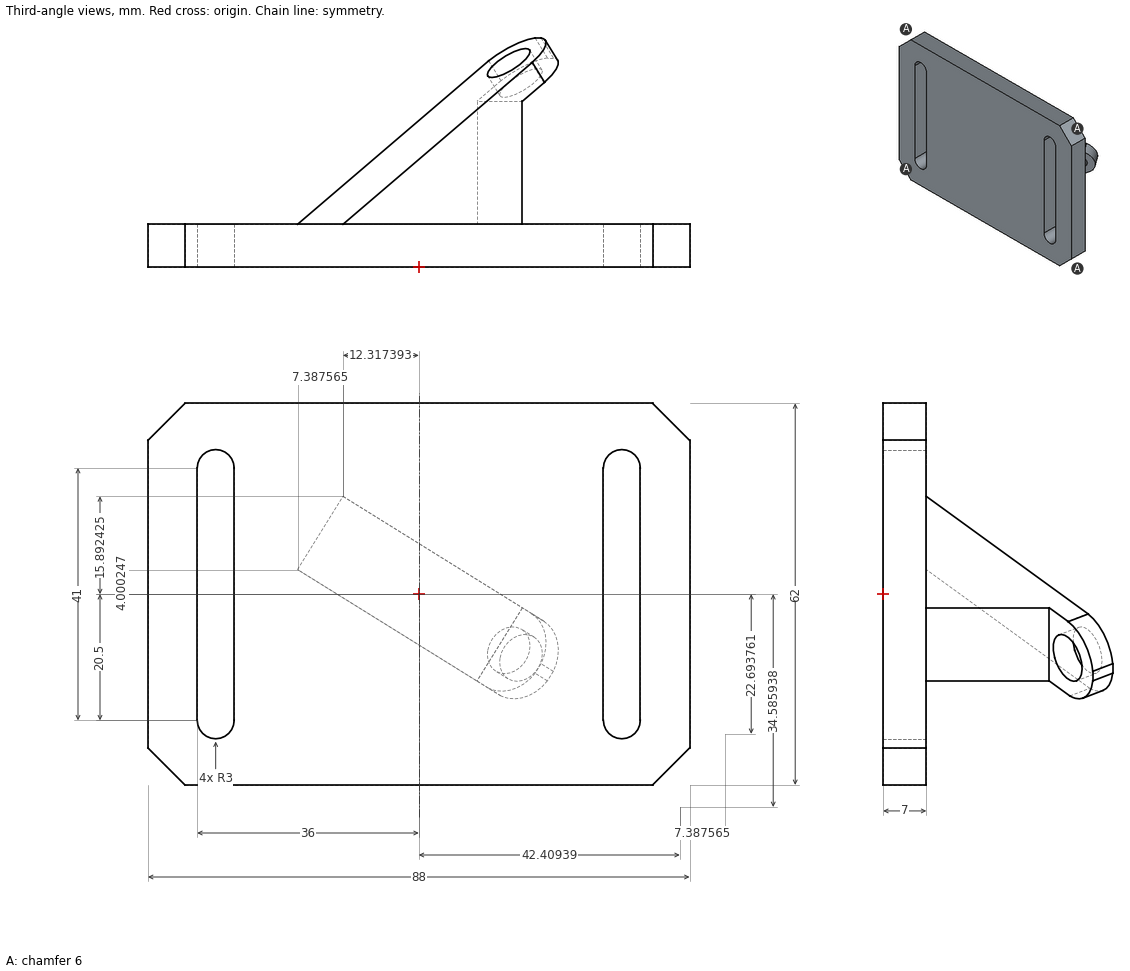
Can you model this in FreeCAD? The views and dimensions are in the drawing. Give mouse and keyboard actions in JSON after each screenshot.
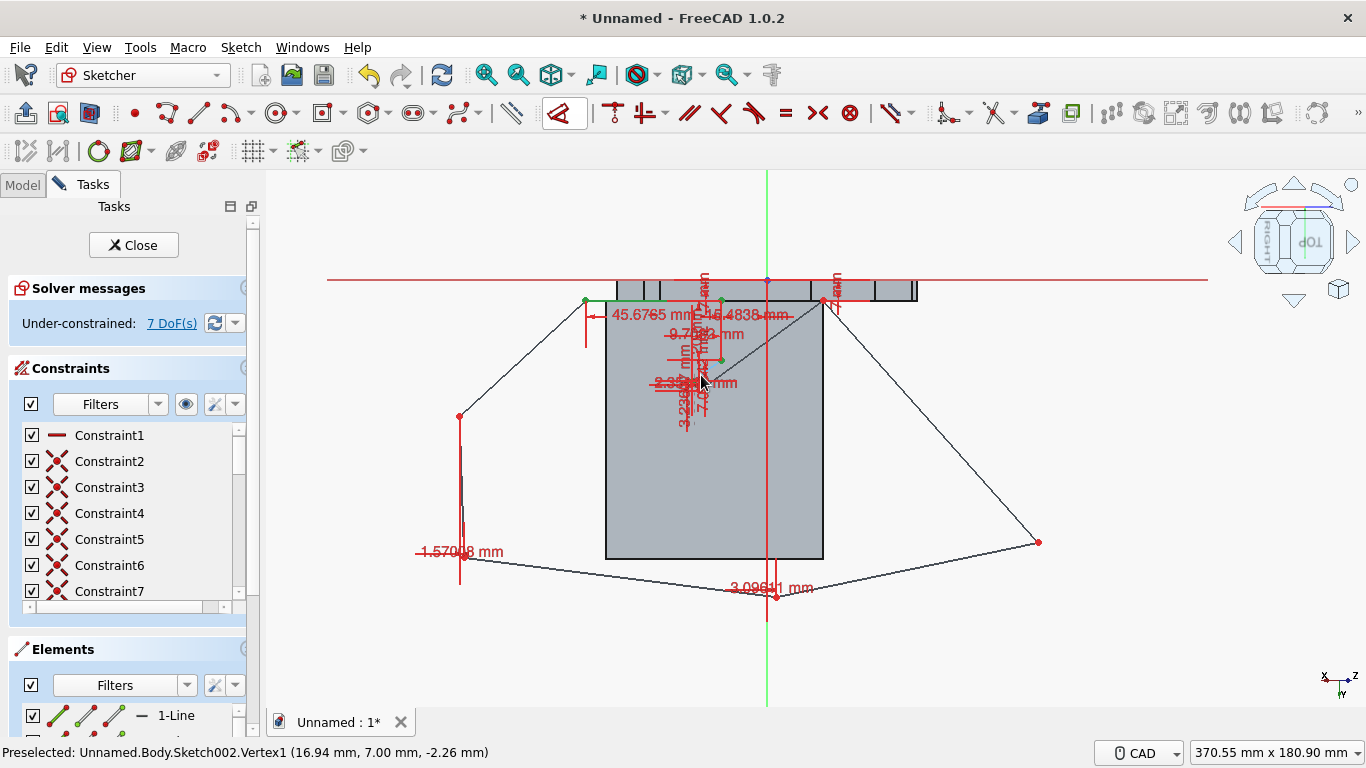
{"action": "left_click", "coordinate": [460, 417]}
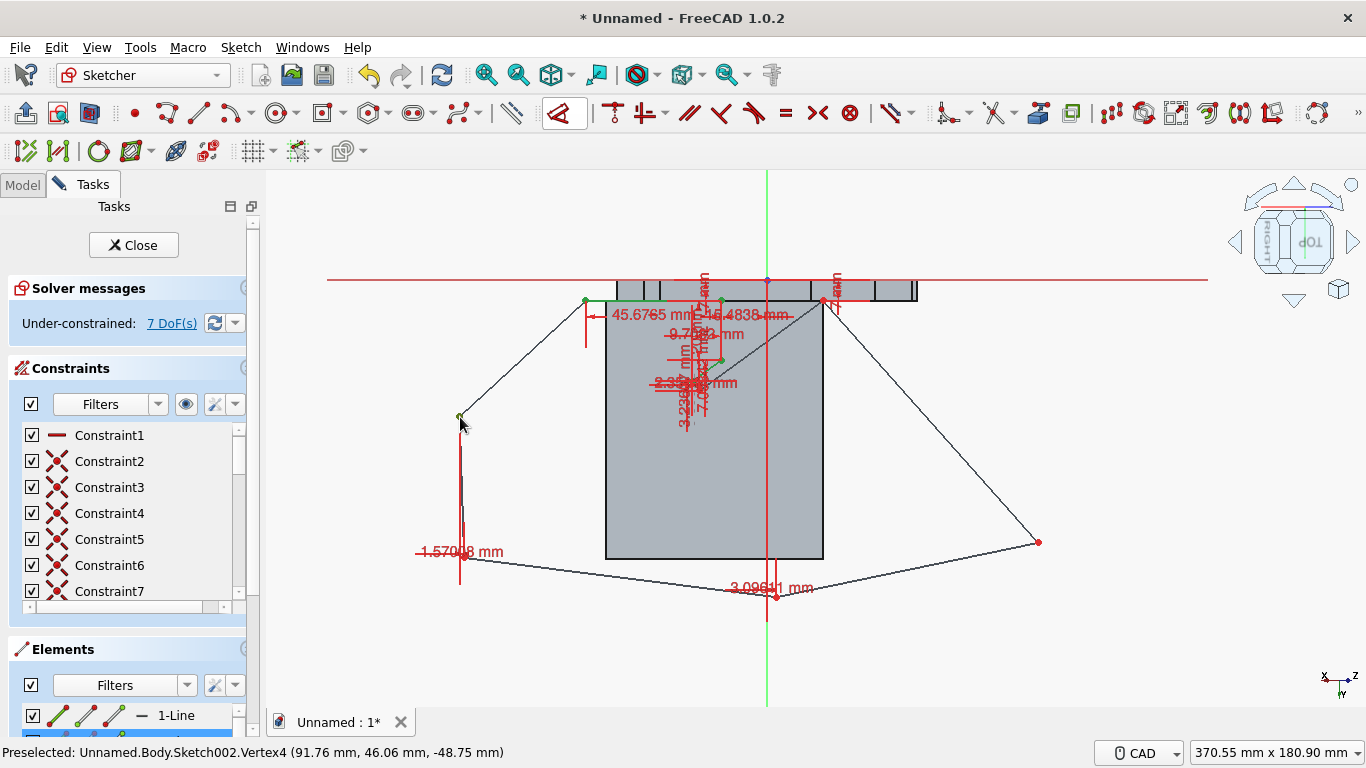
{"action": "left_click", "coordinate": [582, 114]}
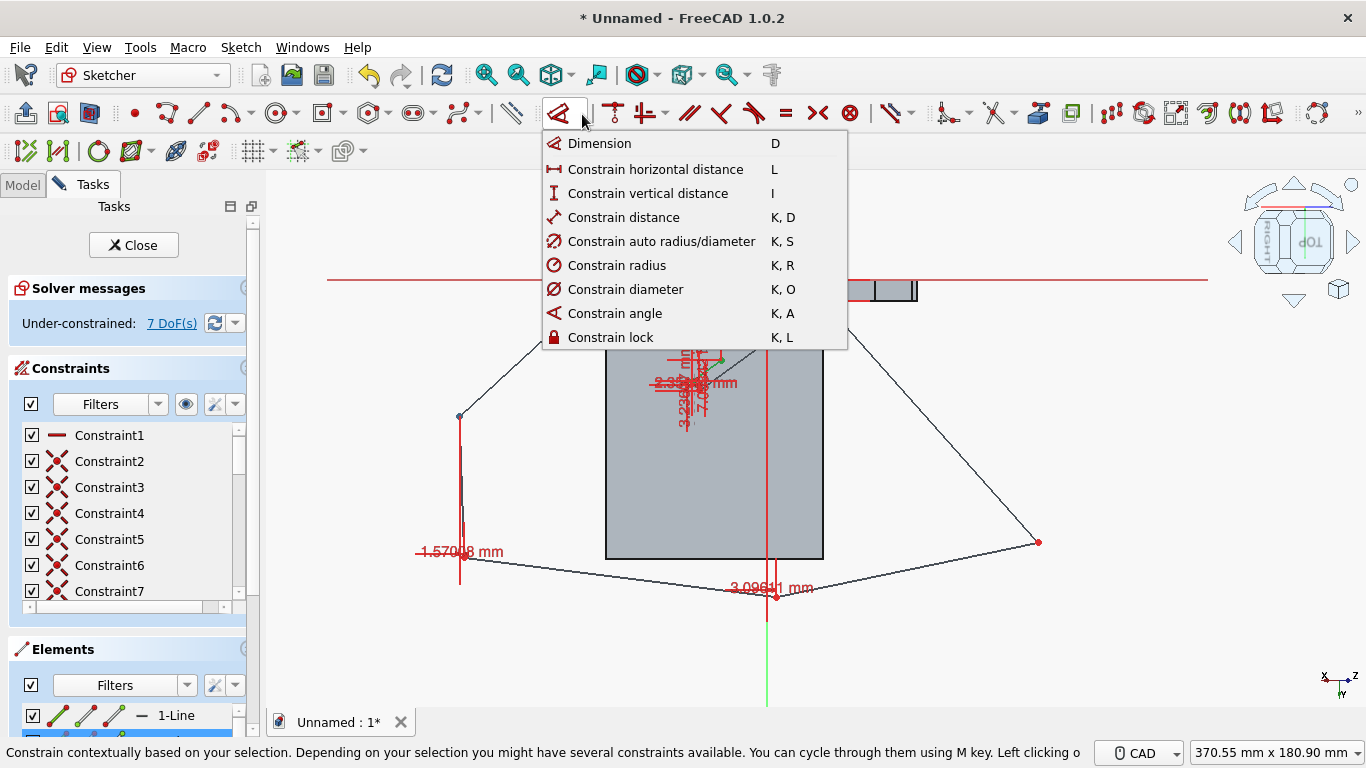
{"action": "left_click", "coordinate": [695, 193]}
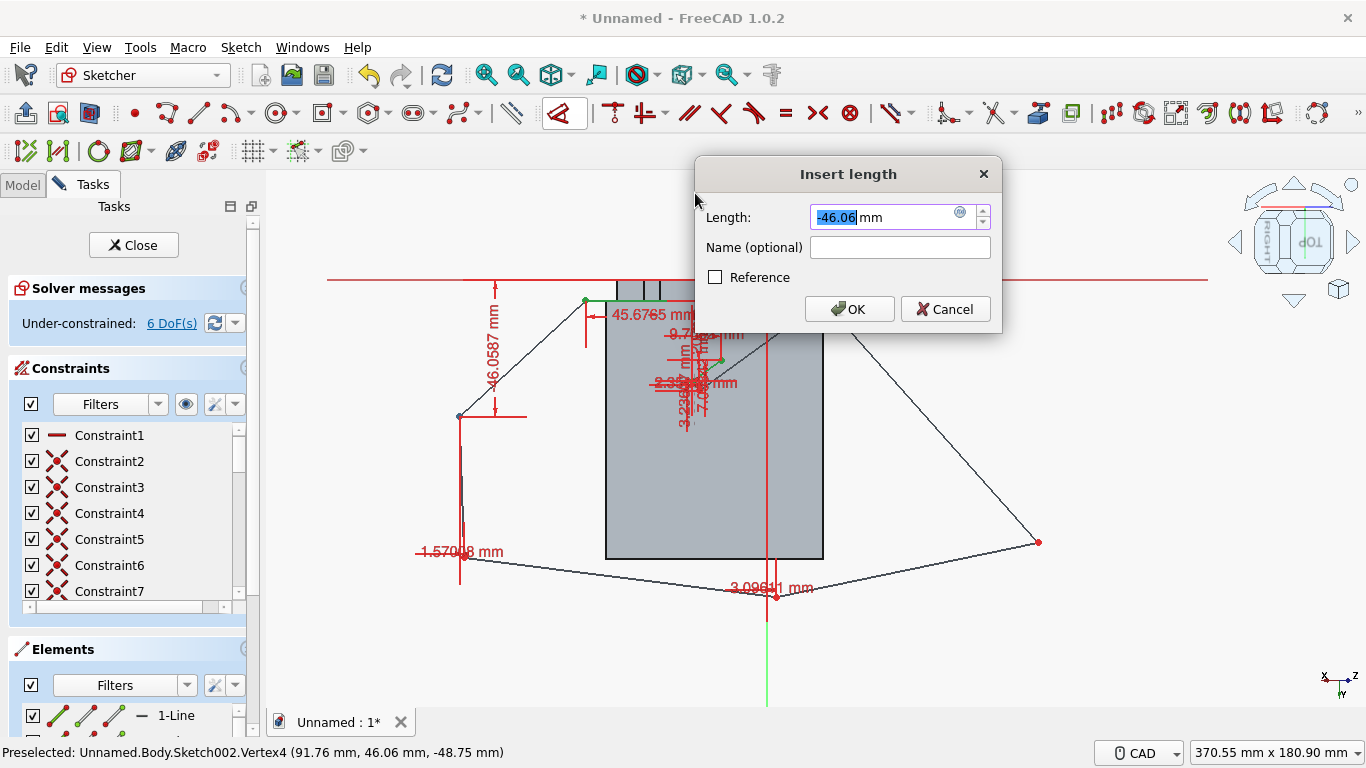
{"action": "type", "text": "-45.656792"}
{"action": "key", "text": "Return"}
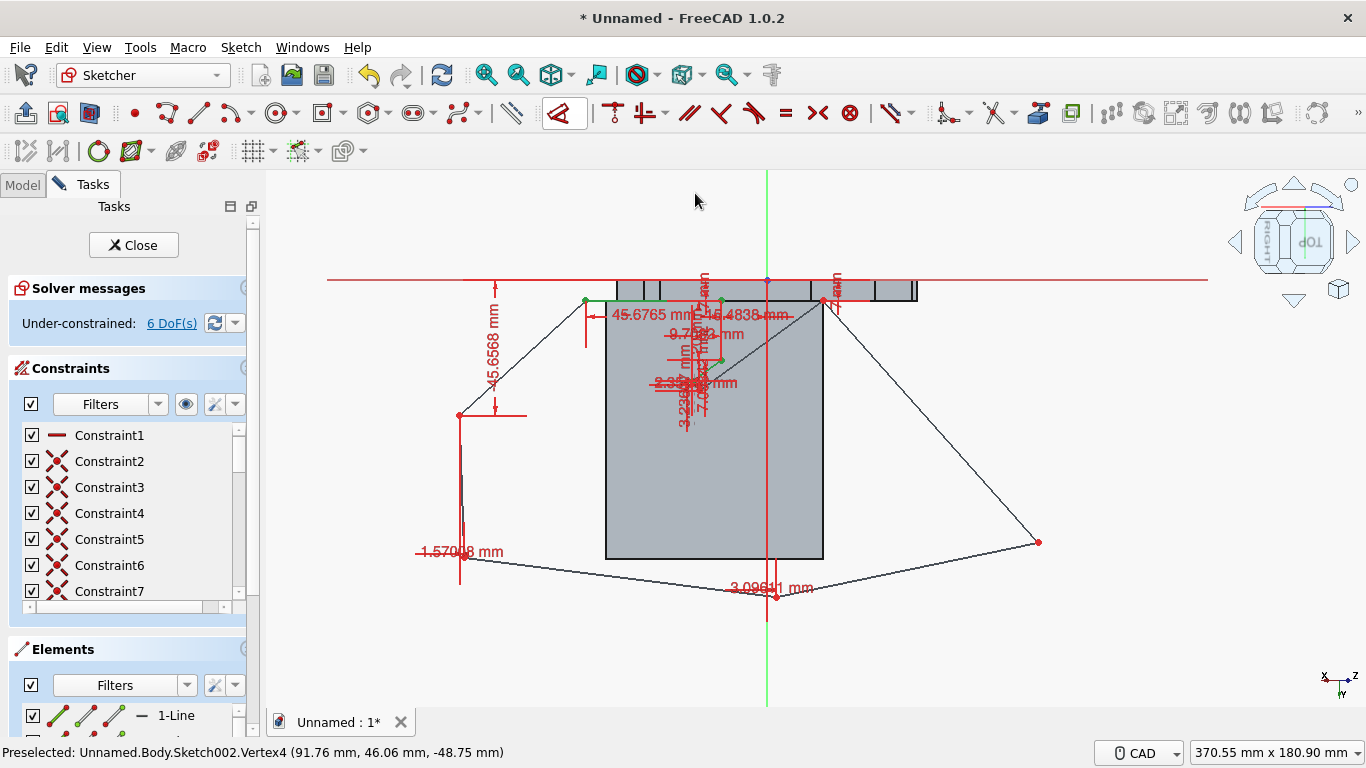
{"action": "left_click", "coordinate": [464, 558]}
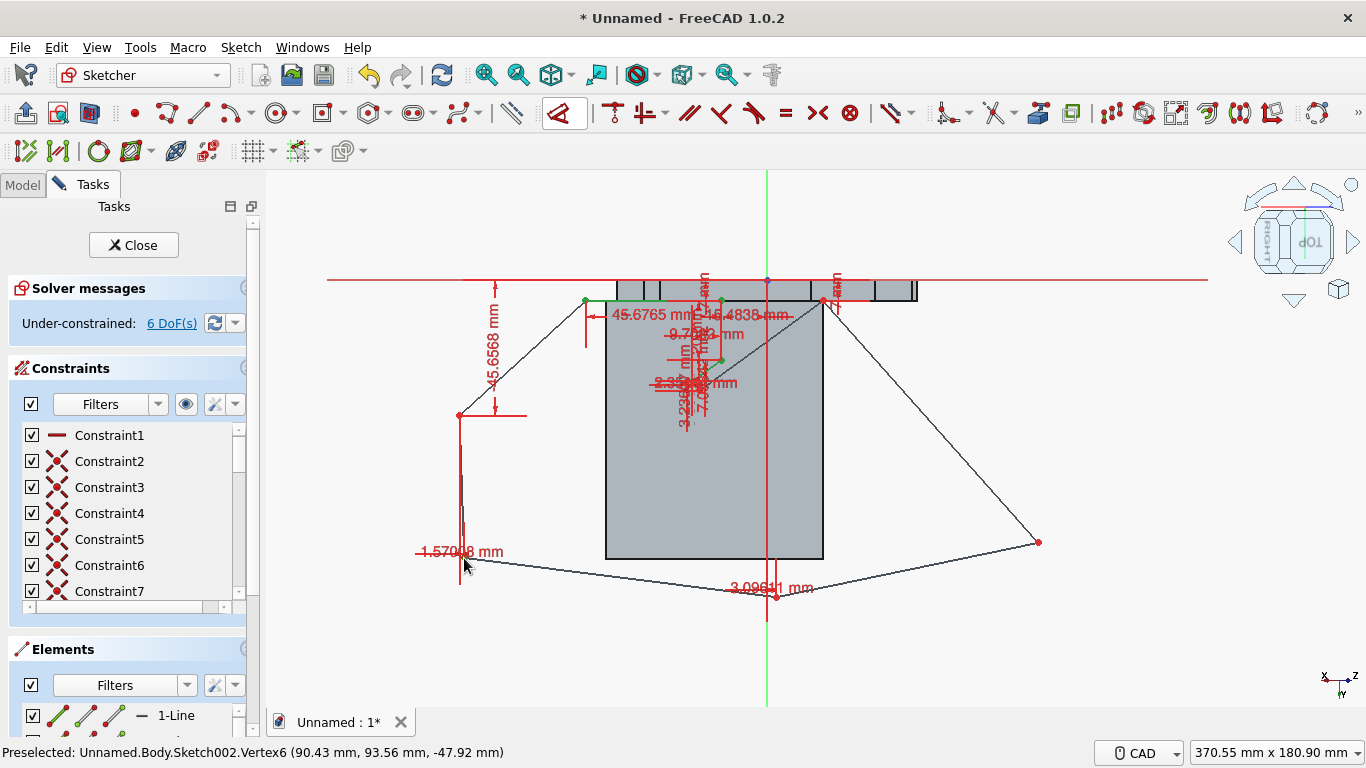
{"action": "left_click", "coordinate": [582, 114]}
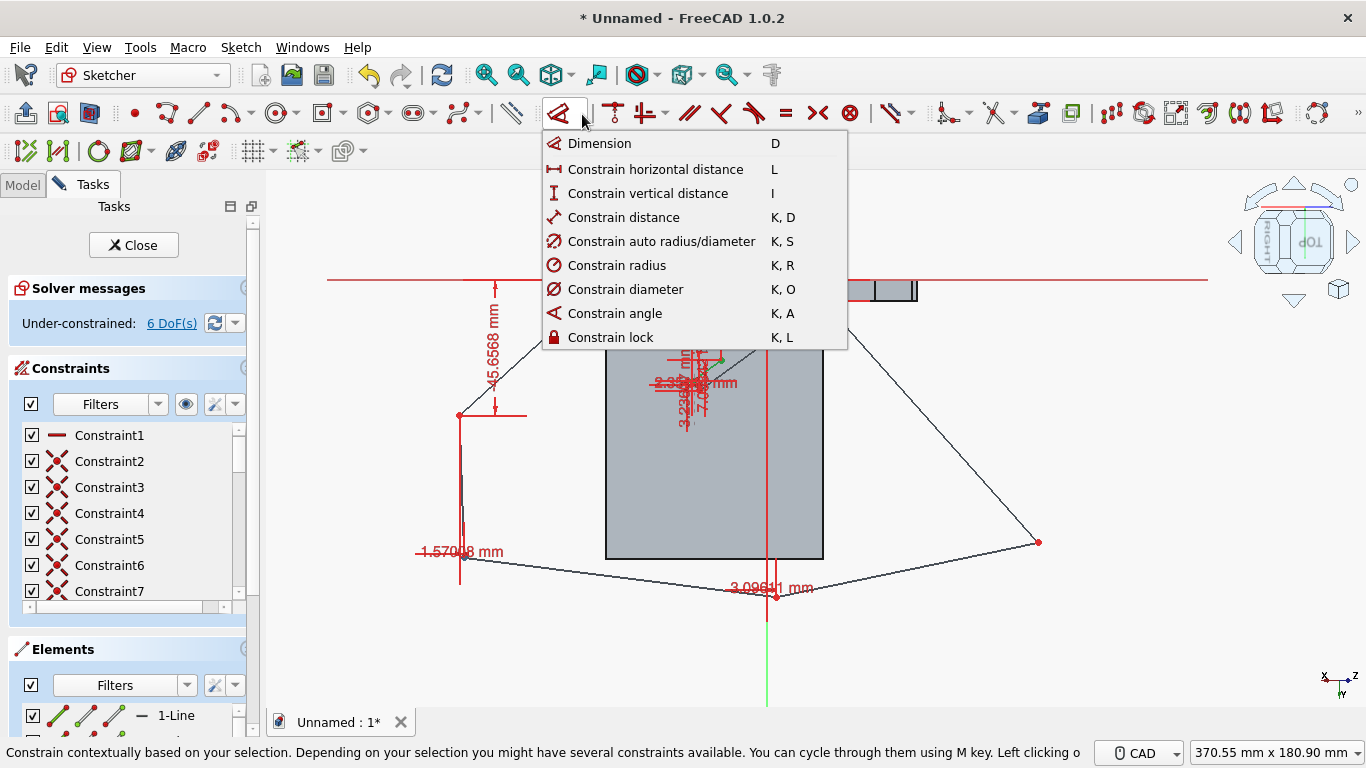
{"action": "left_click", "coordinate": [695, 193]}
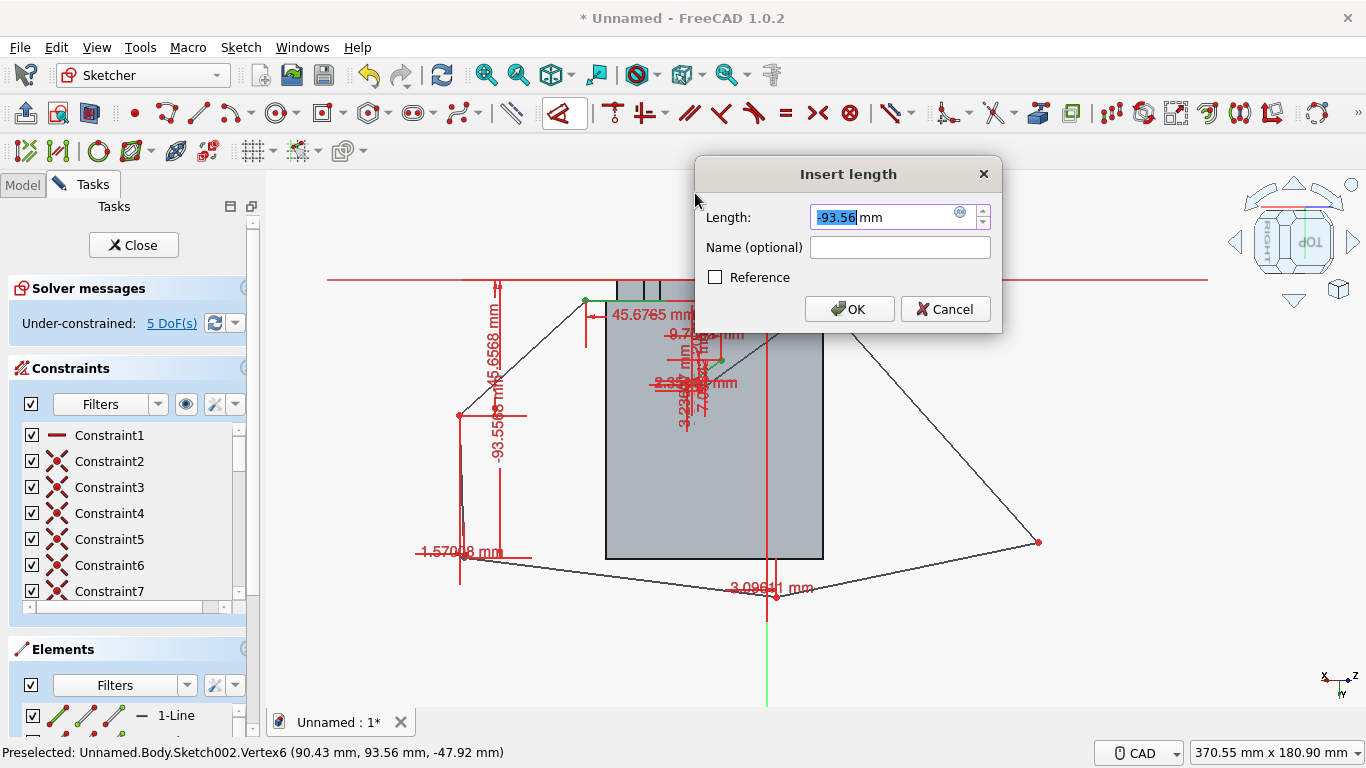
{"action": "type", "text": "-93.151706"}
{"action": "key", "text": "Return"}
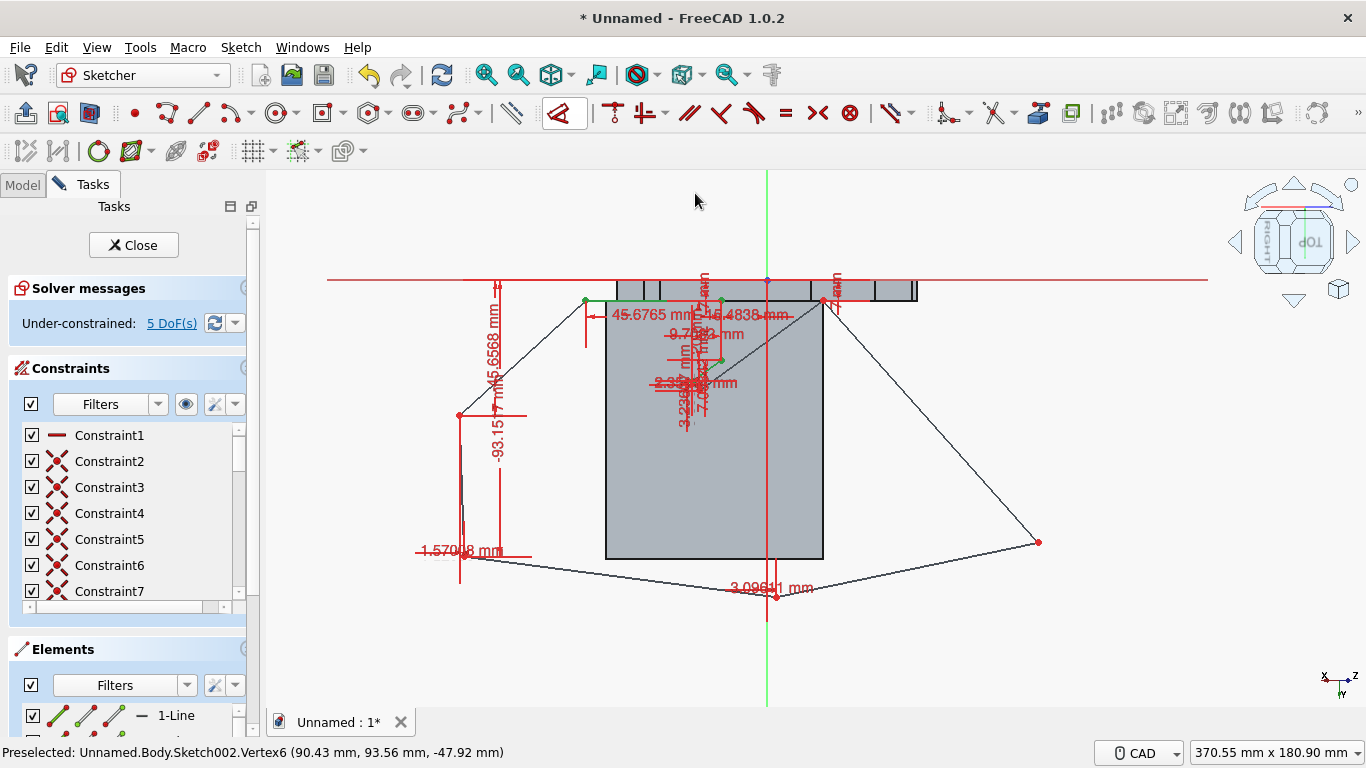
{"action": "left_click", "coordinate": [1038, 543]}